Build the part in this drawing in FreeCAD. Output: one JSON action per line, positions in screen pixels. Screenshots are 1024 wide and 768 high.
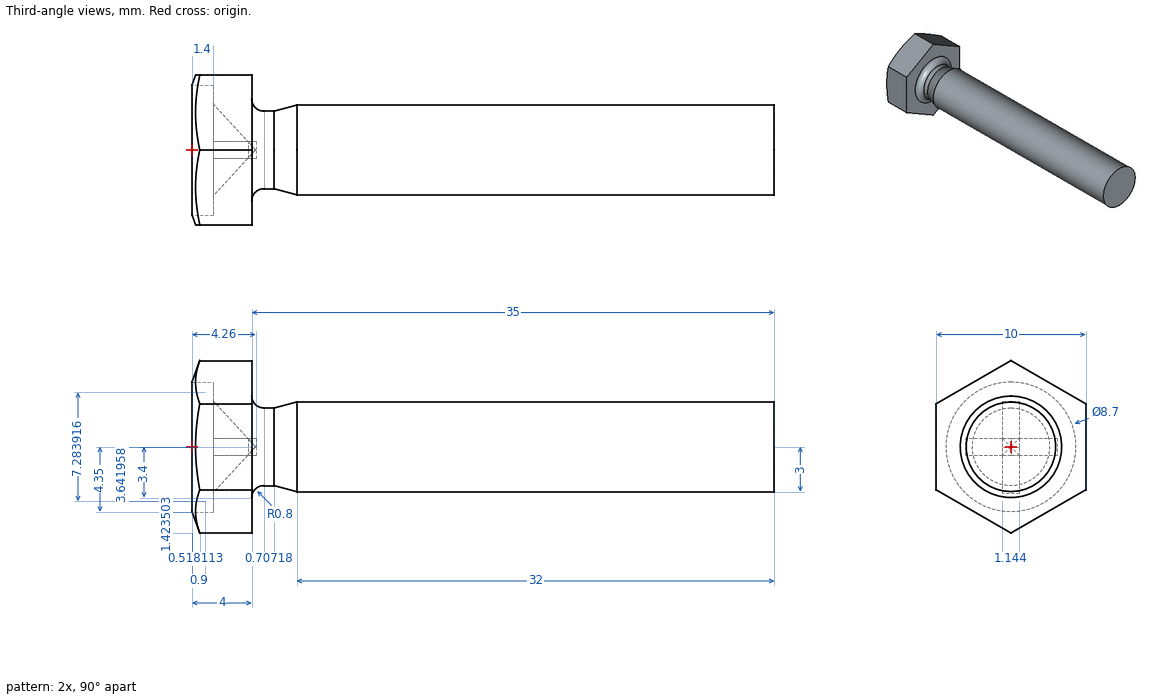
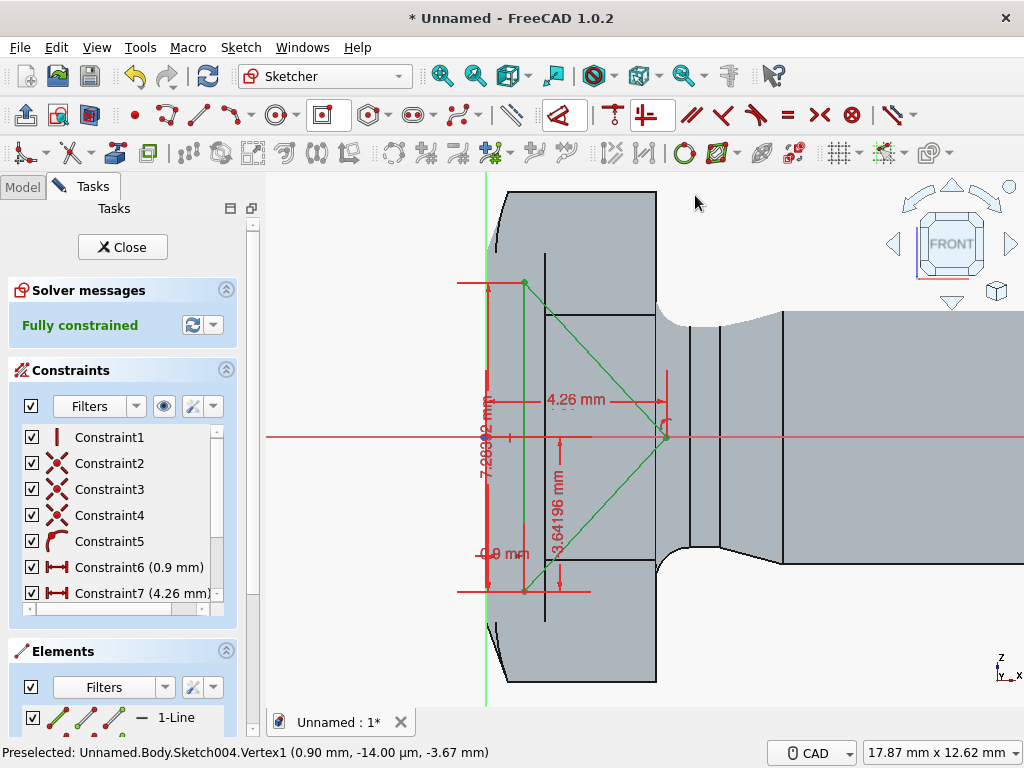
{"action": "left_click", "coordinate": [123, 247]}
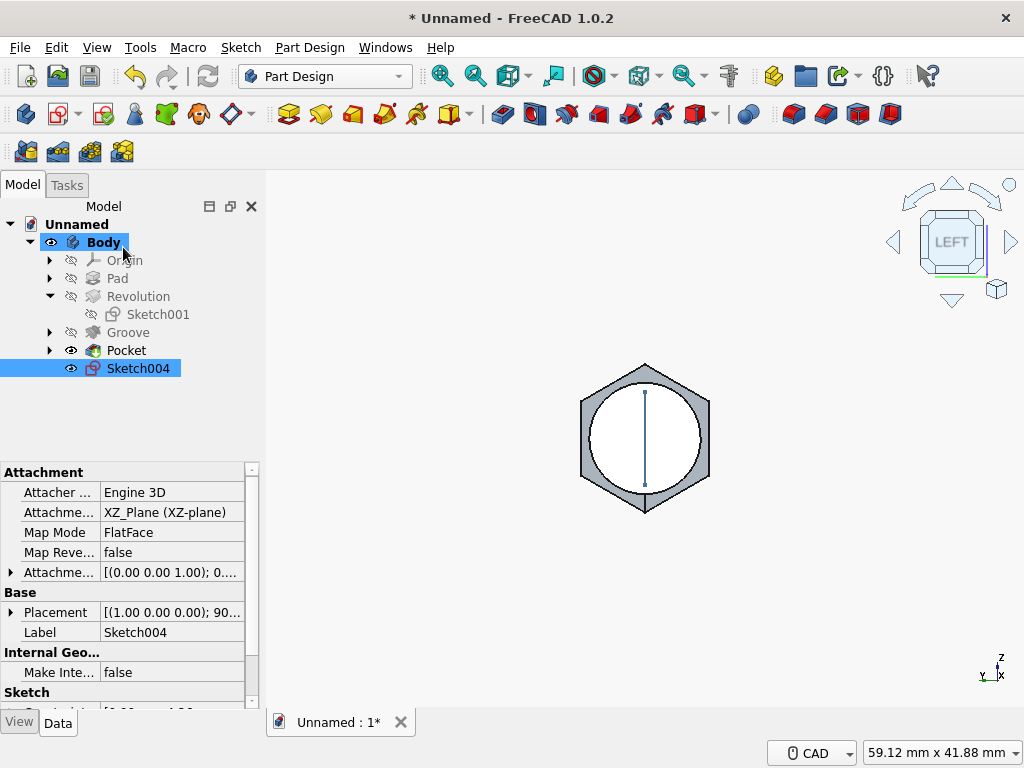
{"action": "left_click", "coordinate": [504, 114]}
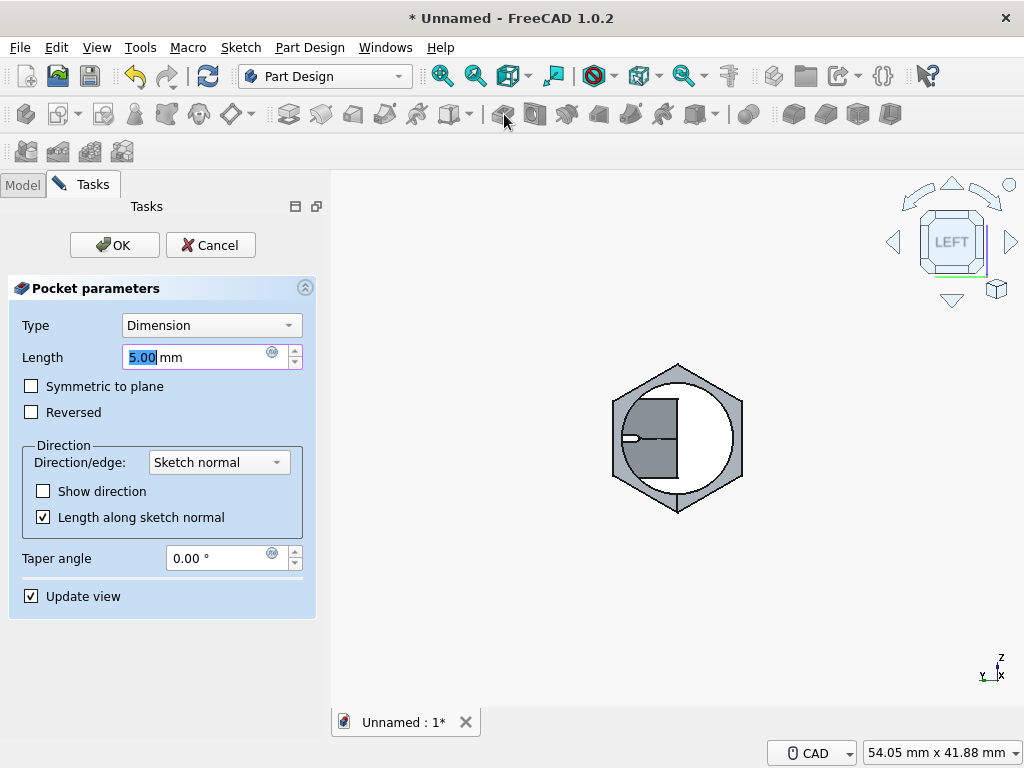
{"action": "type", "text": "1.144"}
{"action": "key", "text": "Tab"}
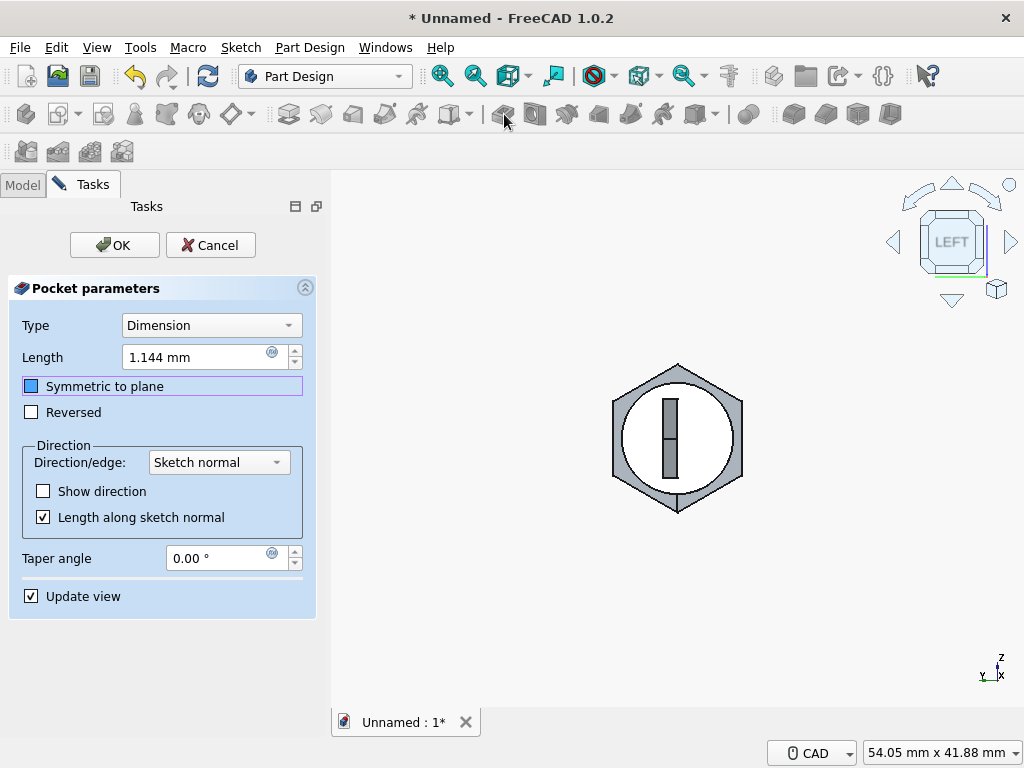
{"action": "left_click", "coordinate": [30, 386]}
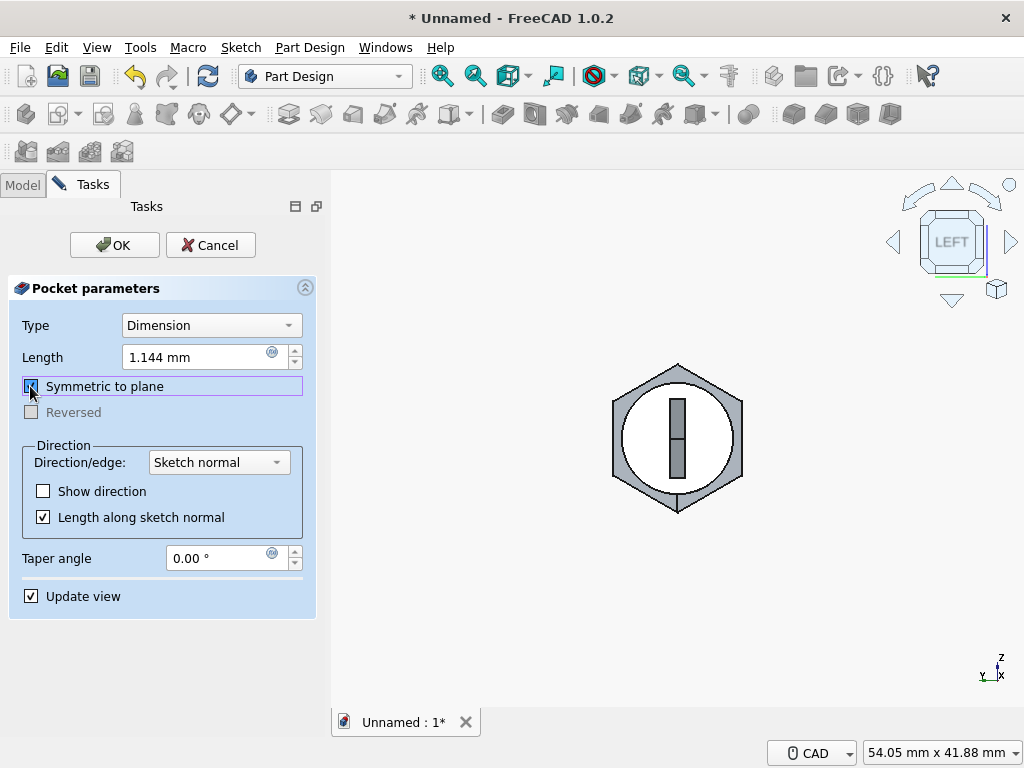
{"action": "left_click", "coordinate": [115, 245]}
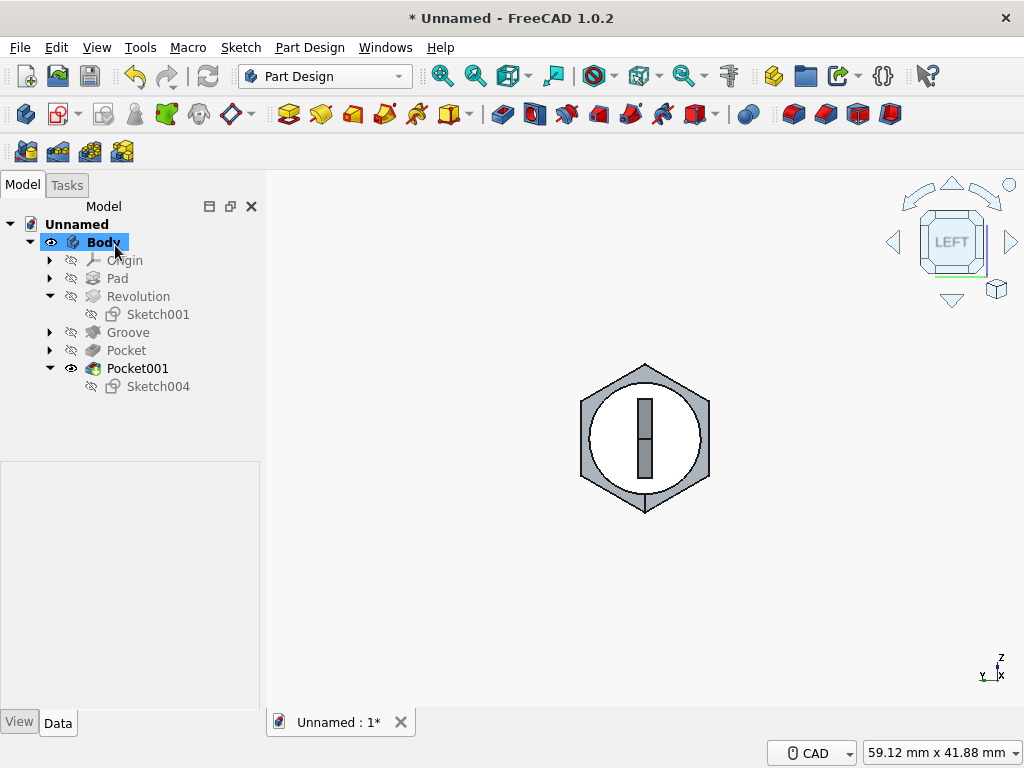
{"action": "key", "text": "v f"}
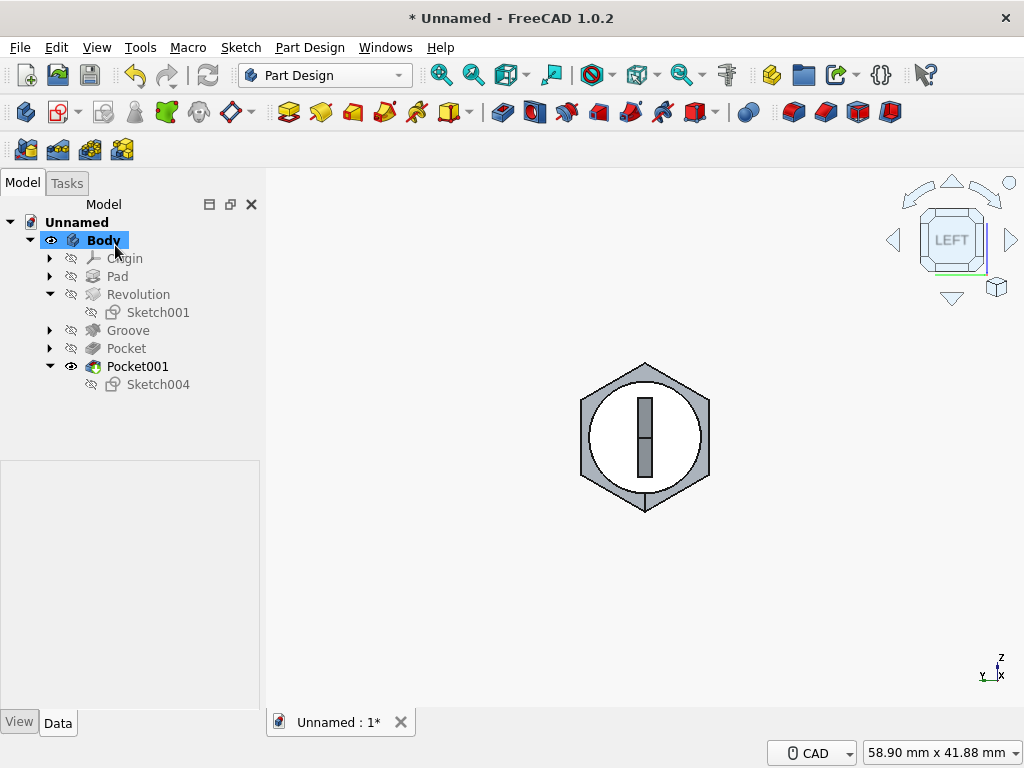
{"action": "left_click", "coordinate": [116, 366]}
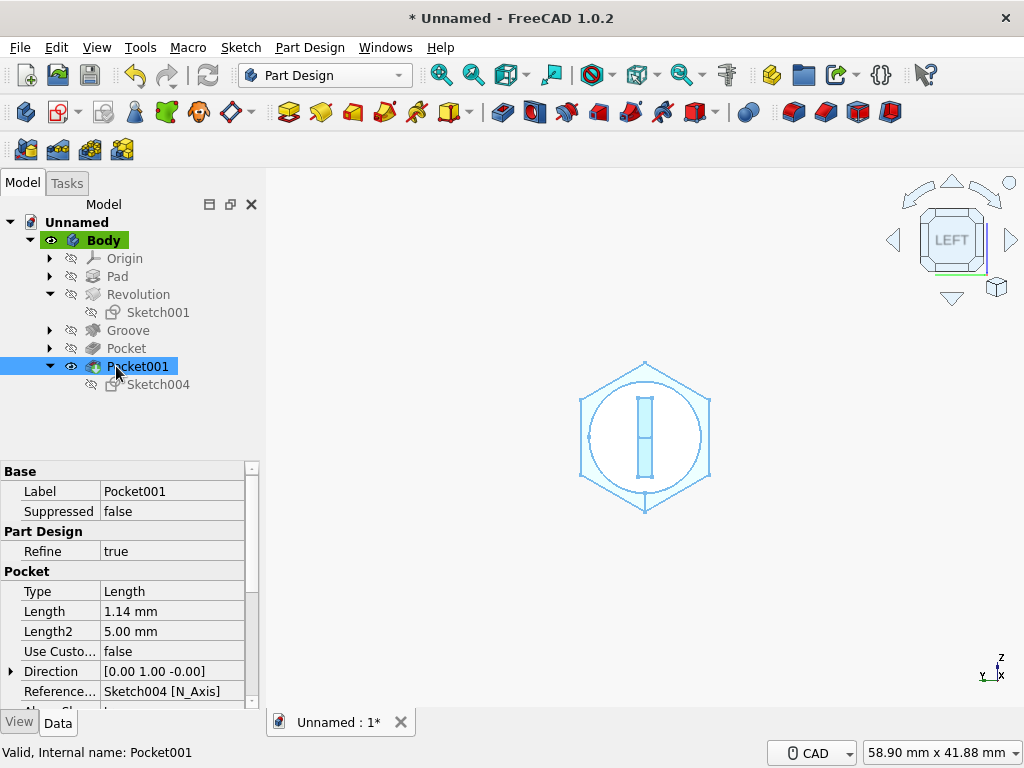
{"action": "left_click", "coordinate": [90, 150]}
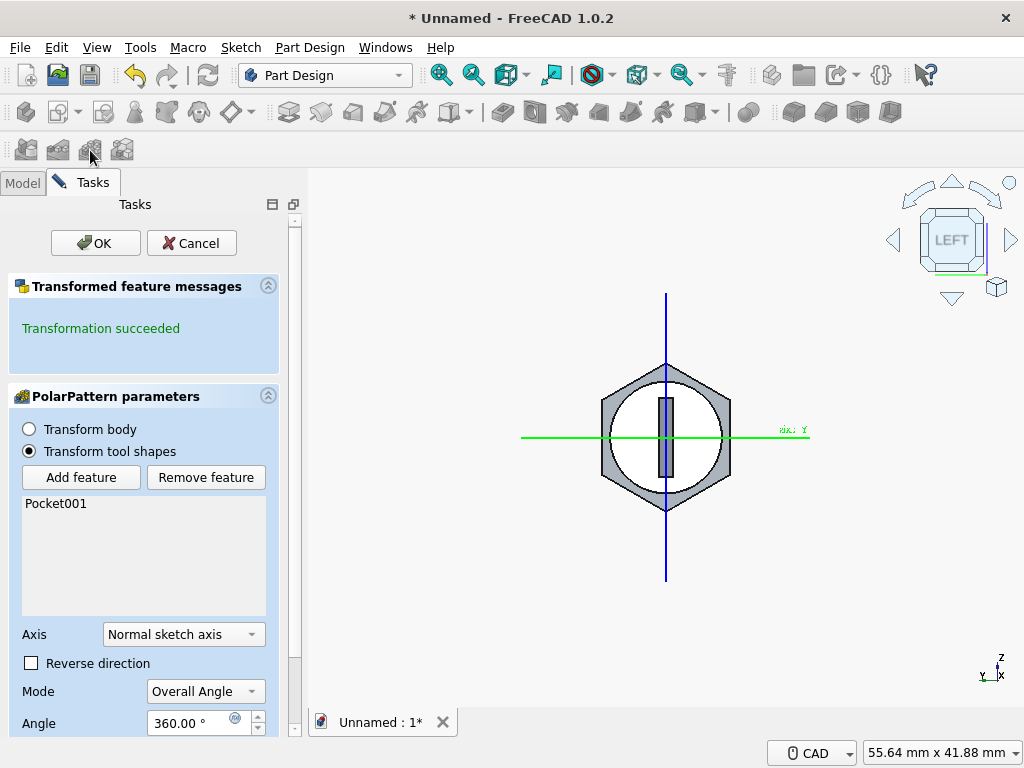
{"action": "left_click", "coordinate": [184, 634]}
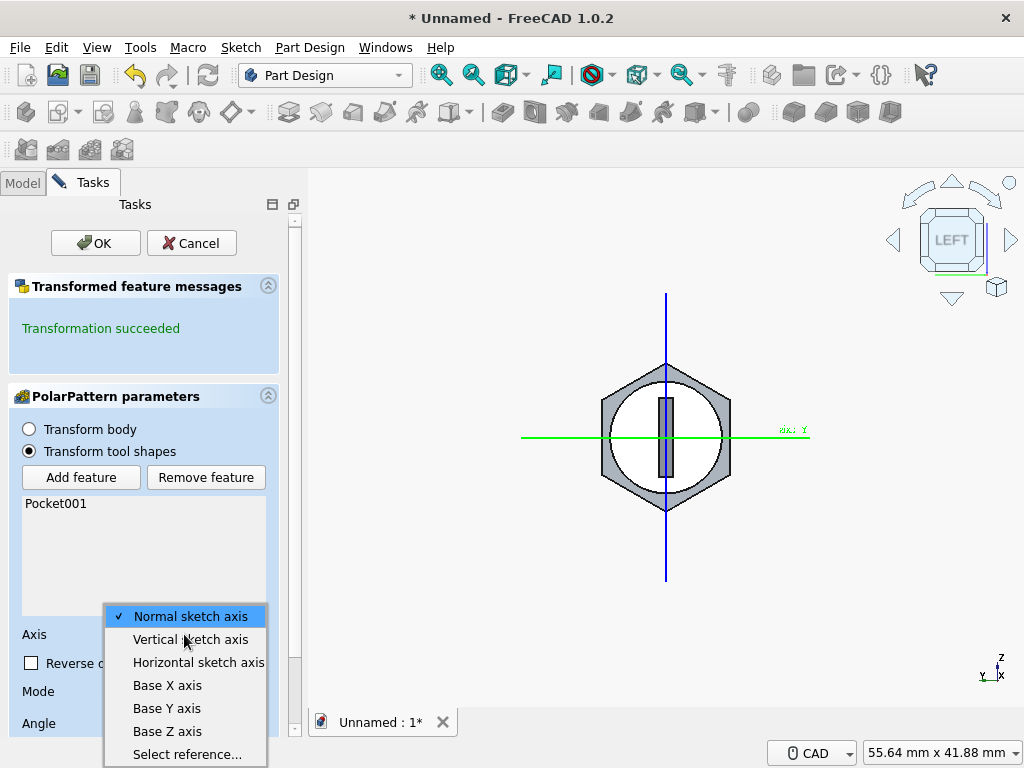
{"action": "left_click", "coordinate": [184, 686]}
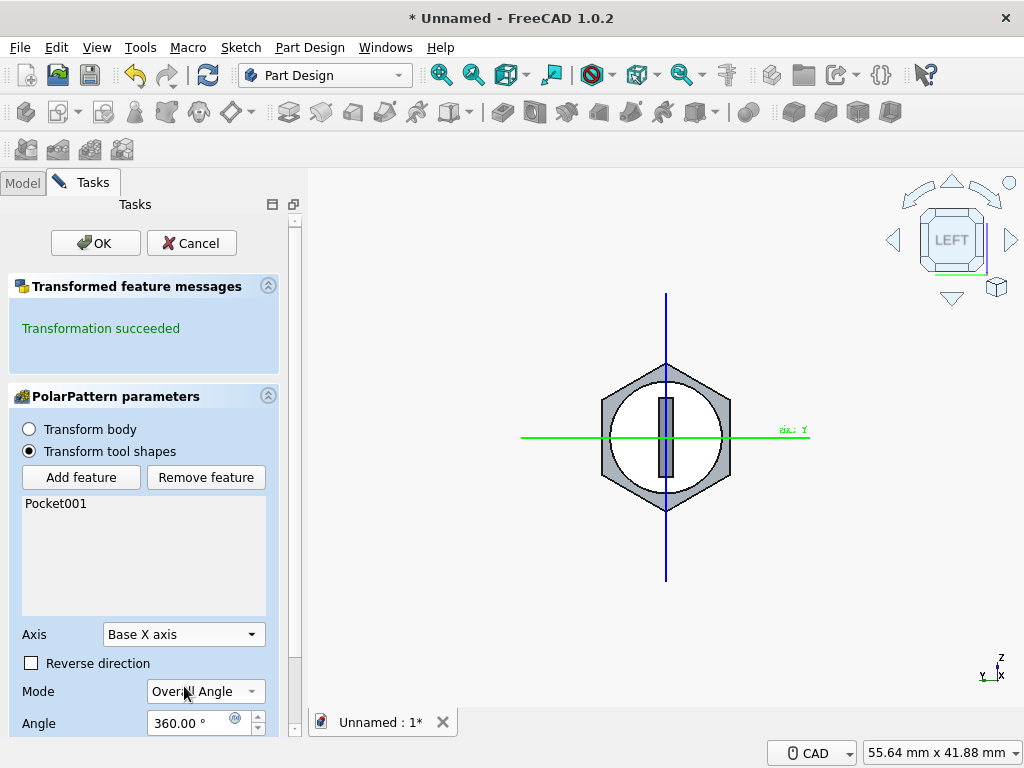
{"action": "left_click", "coordinate": [206, 692]}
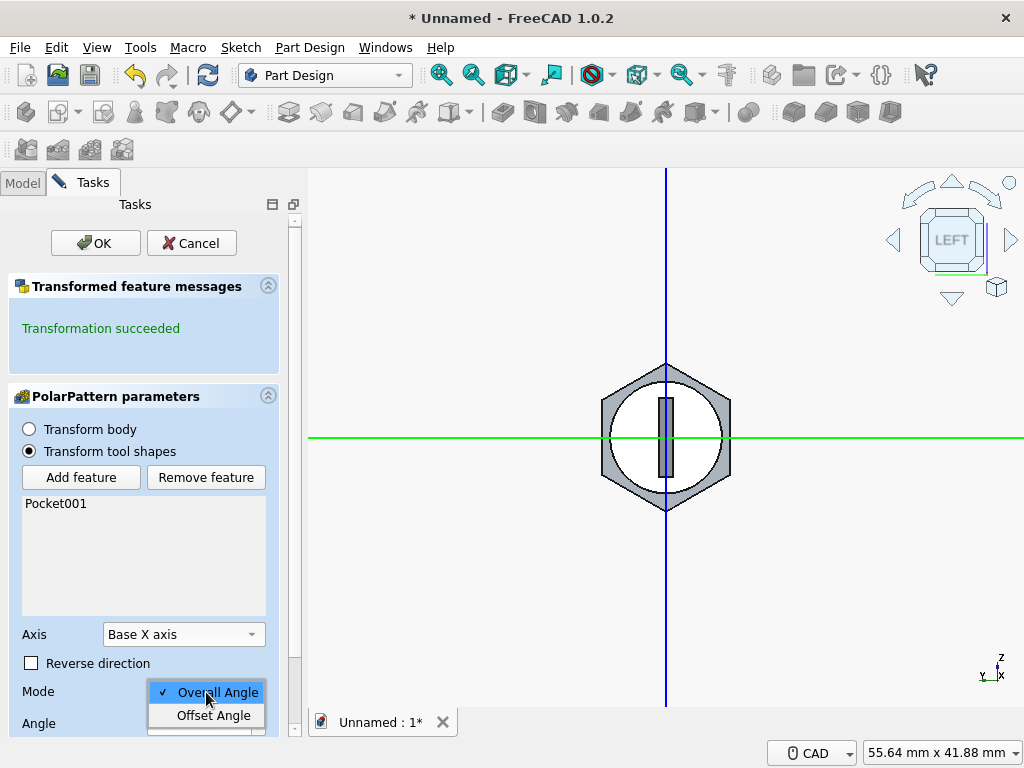
{"action": "left_click", "coordinate": [206, 716]}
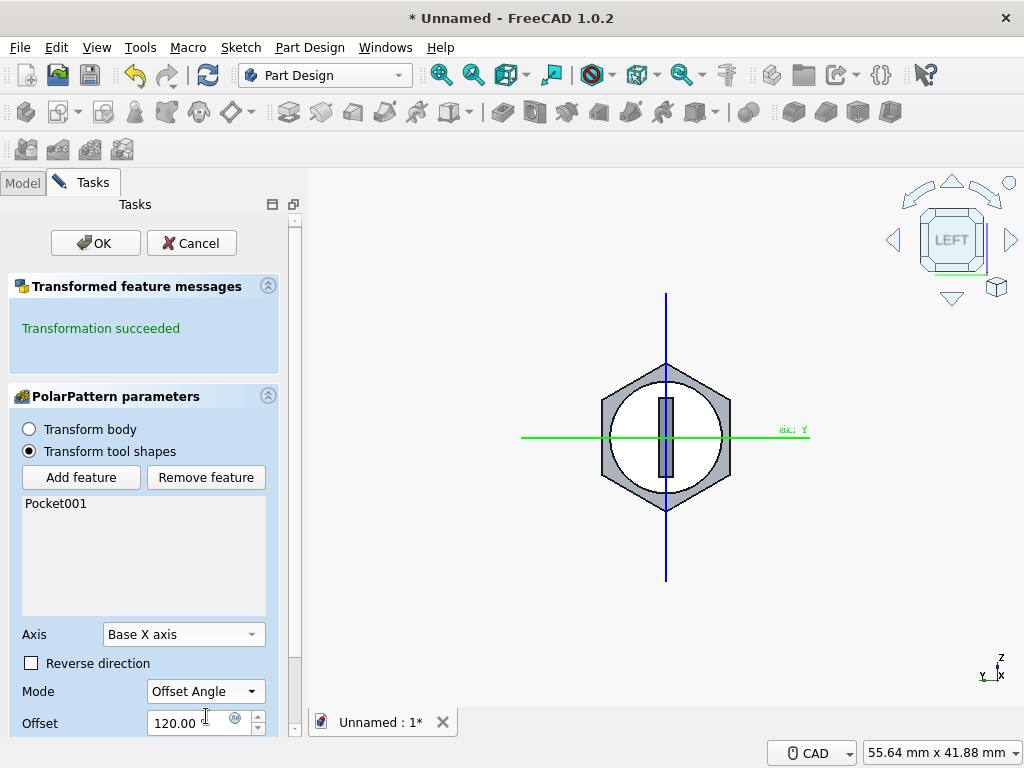
{"action": "triple_click", "coordinate": [198, 723]}